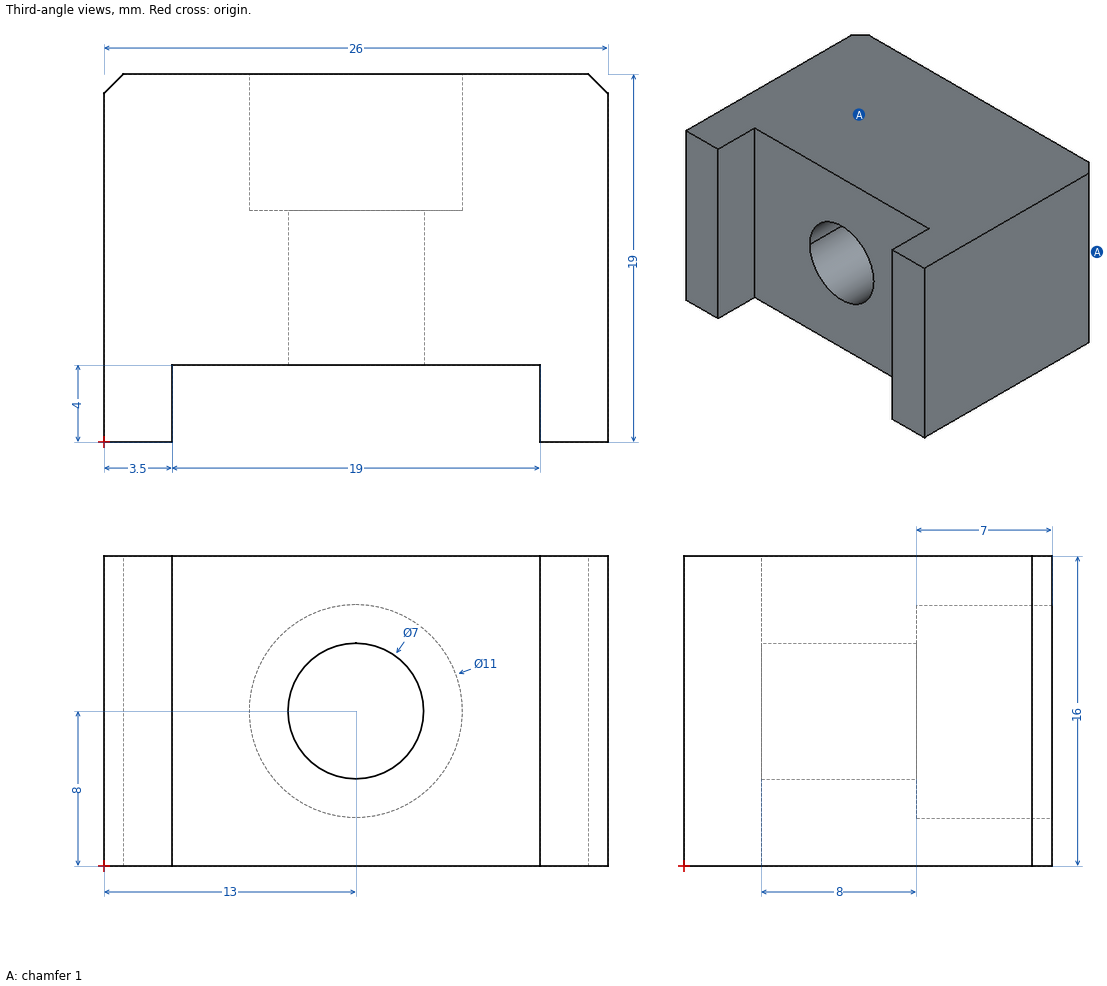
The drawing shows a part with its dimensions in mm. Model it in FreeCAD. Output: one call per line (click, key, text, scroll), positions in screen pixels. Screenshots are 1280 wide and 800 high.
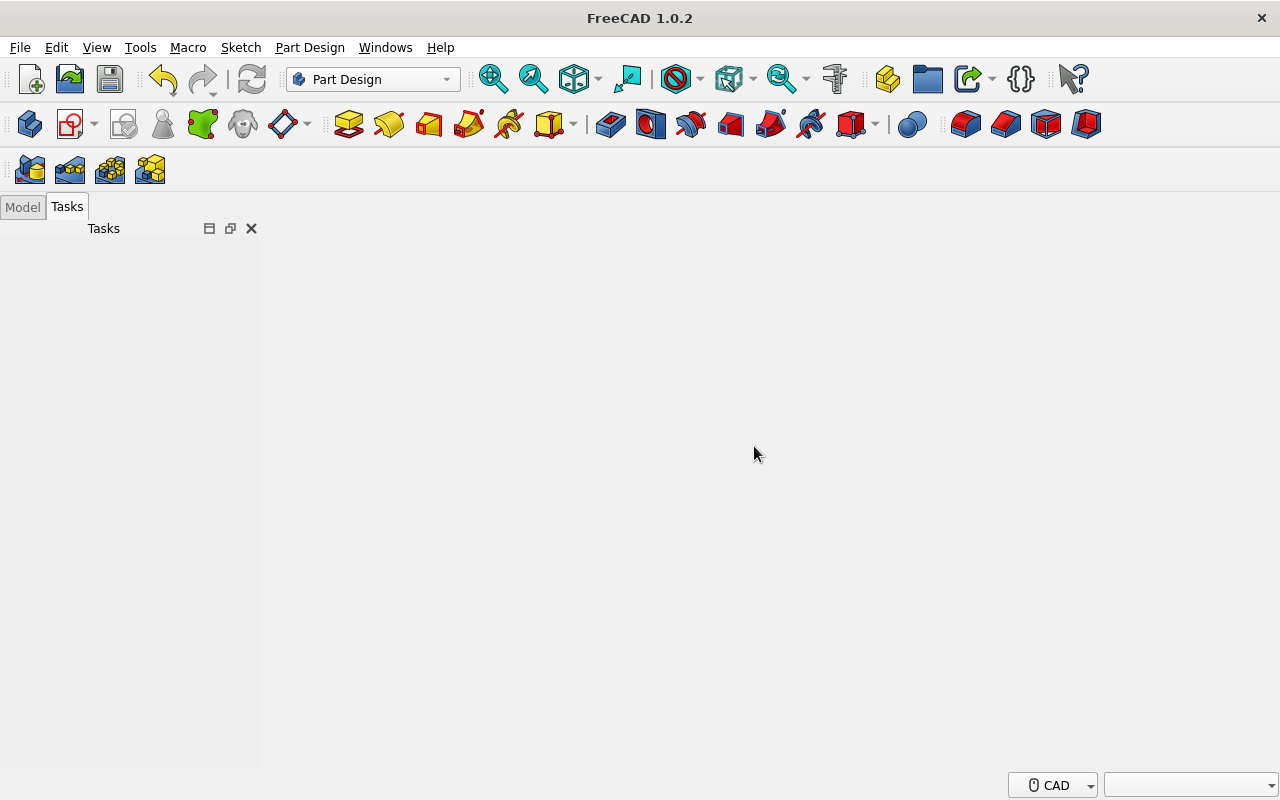
key(ctrl+n)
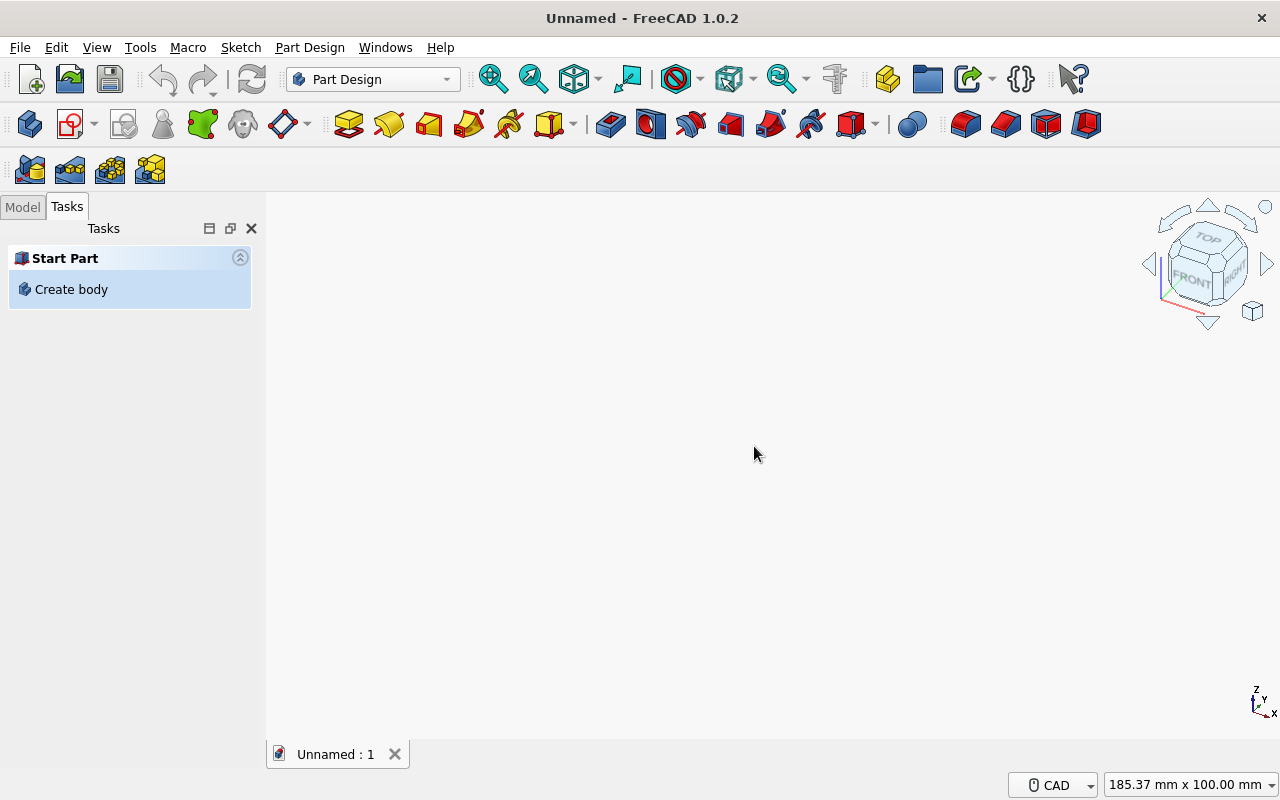
click(70, 124)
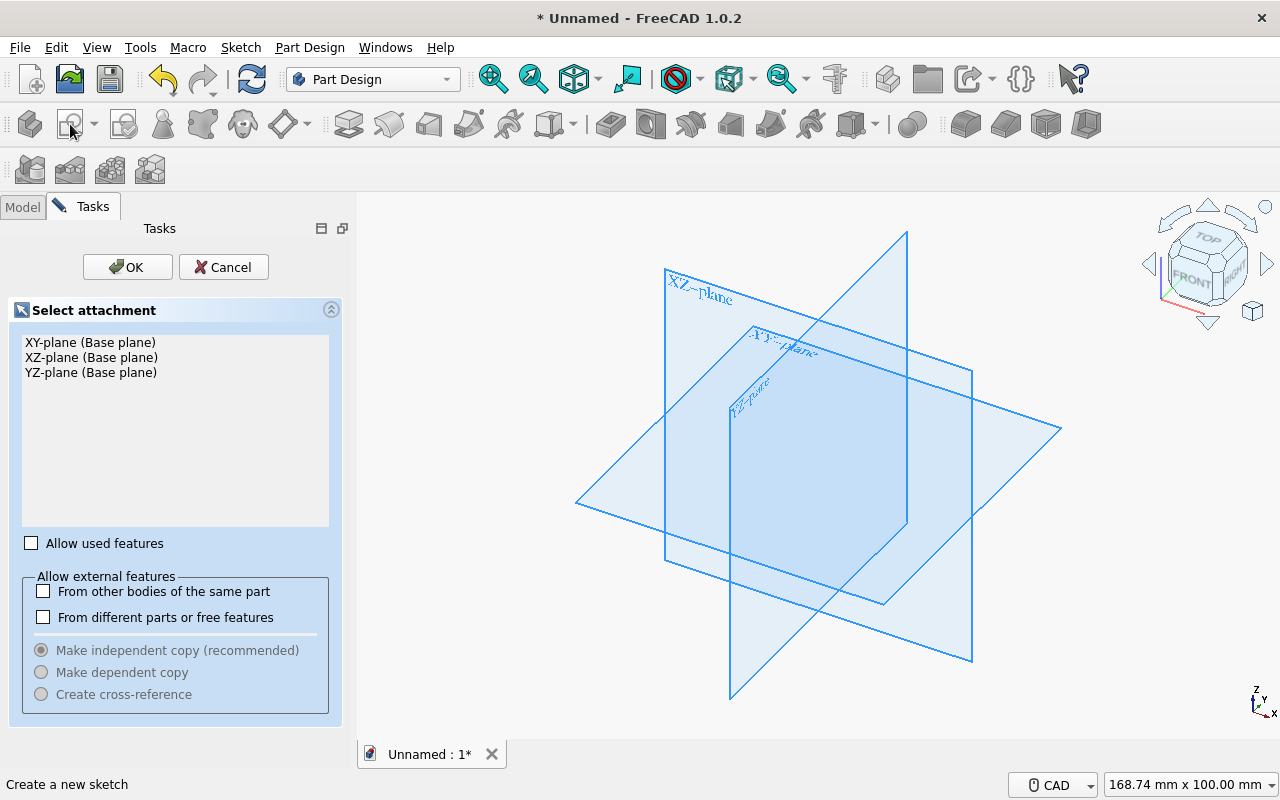
click(82, 342)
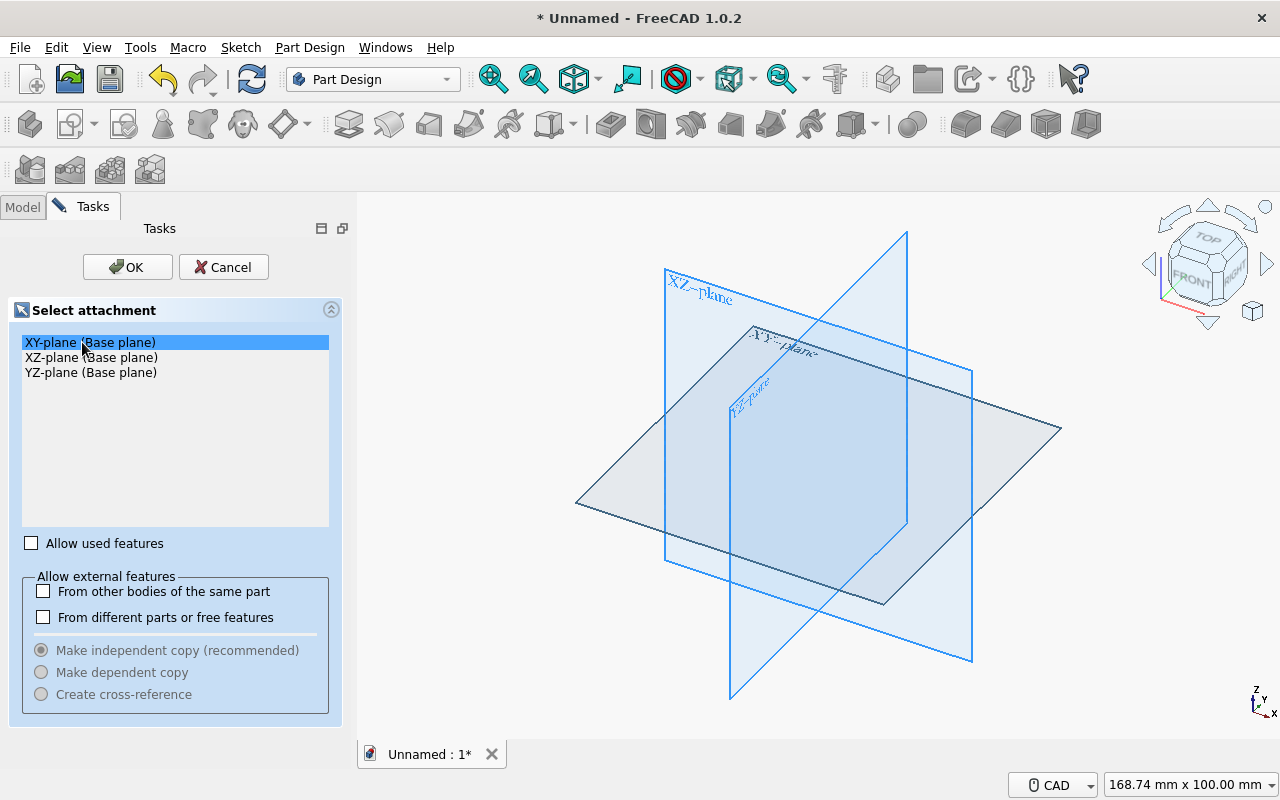
click(128, 267)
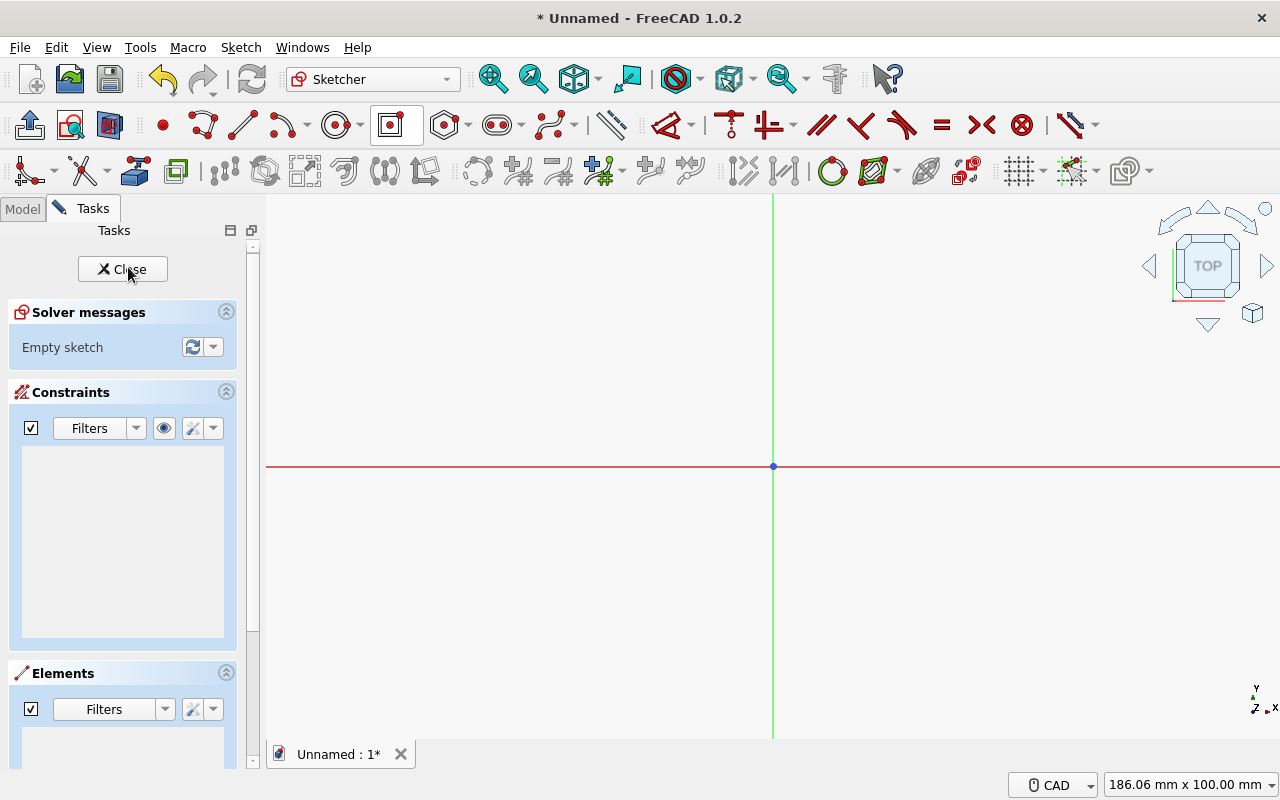
scroll(904, 392, up, 6)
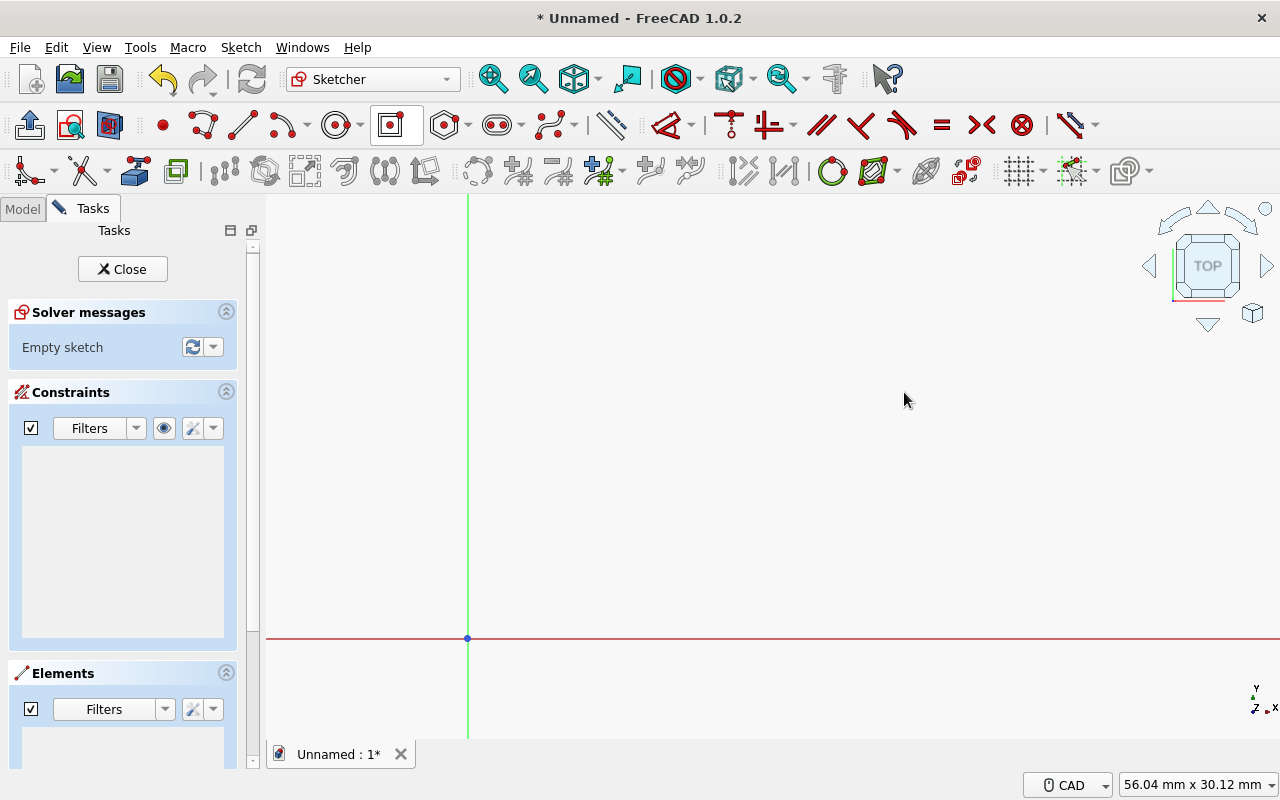
click(204, 126)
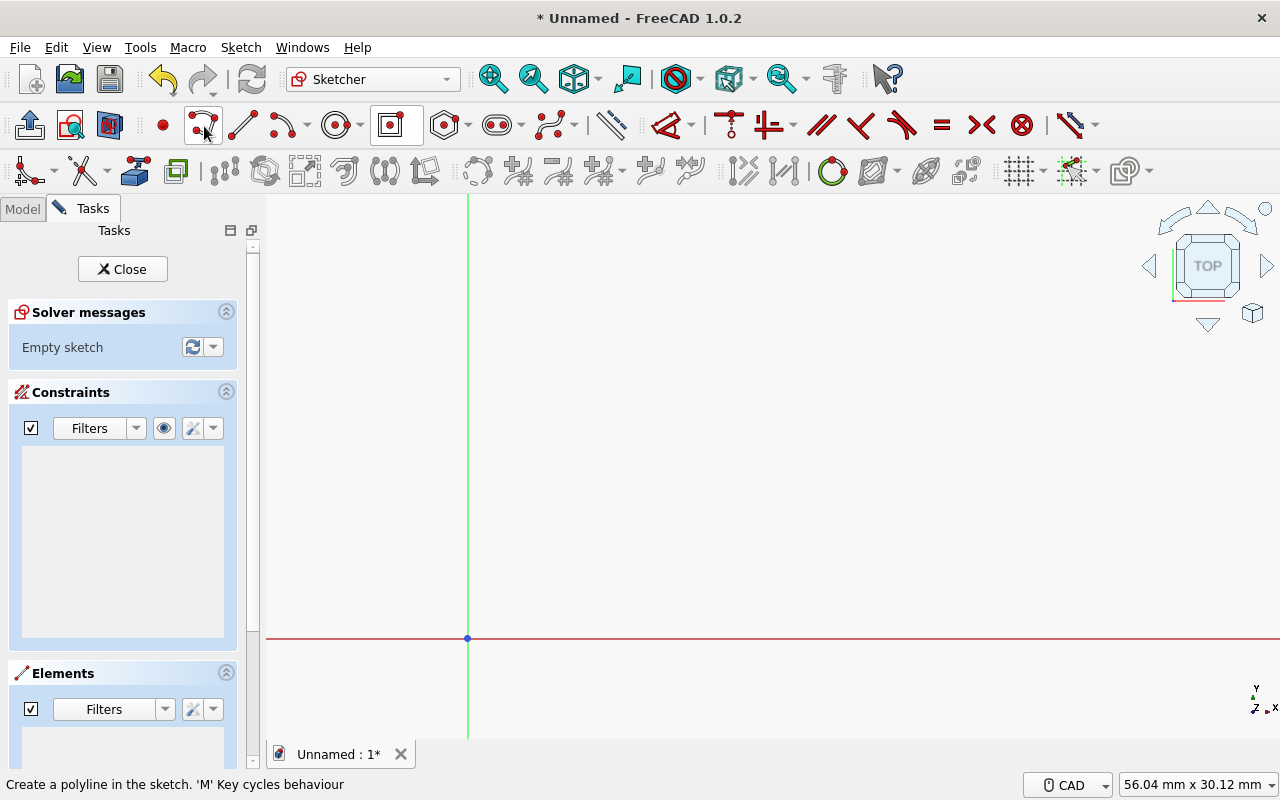
click(468, 639)
click(531, 630)
click(531, 566)
click(875, 566)
click(875, 639)
click(938, 630)
click(938, 295)
click(477, 295)
click(468, 639)
key(Escape)
key(Escape)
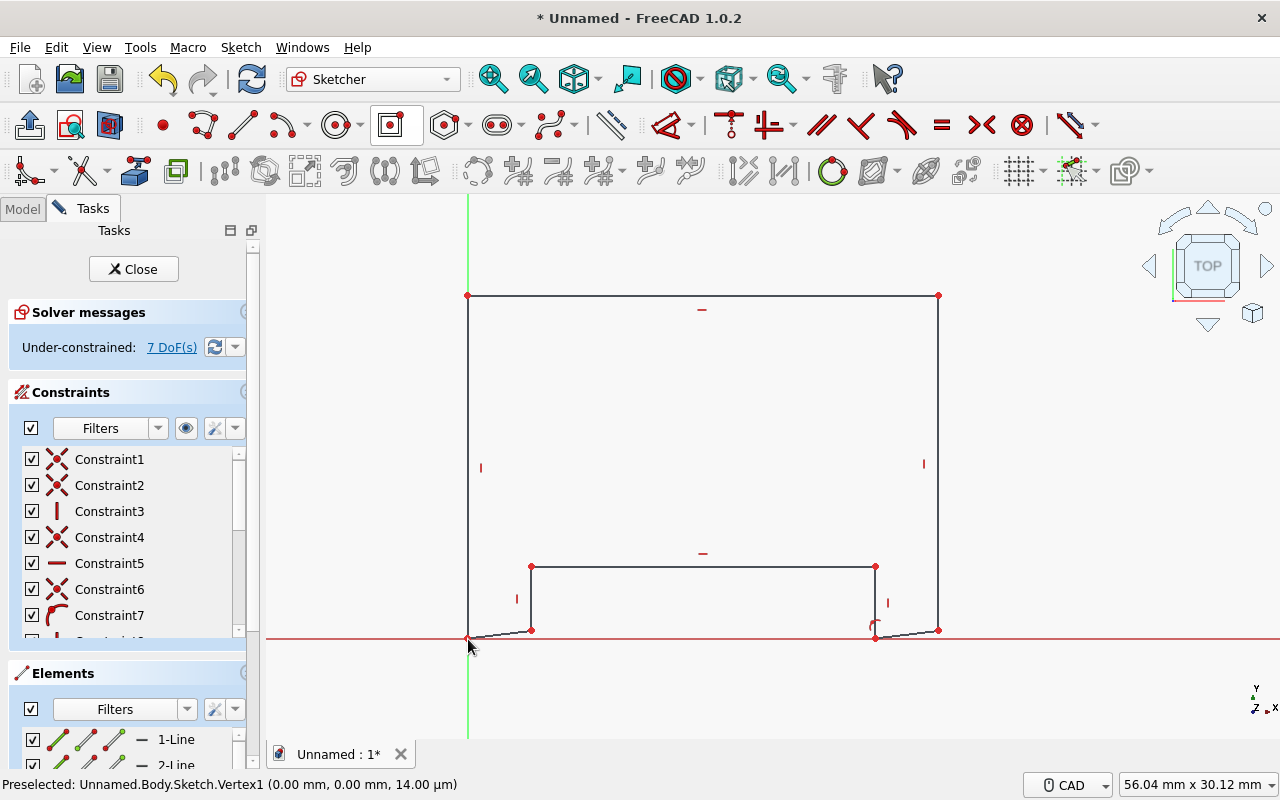
click(487, 636)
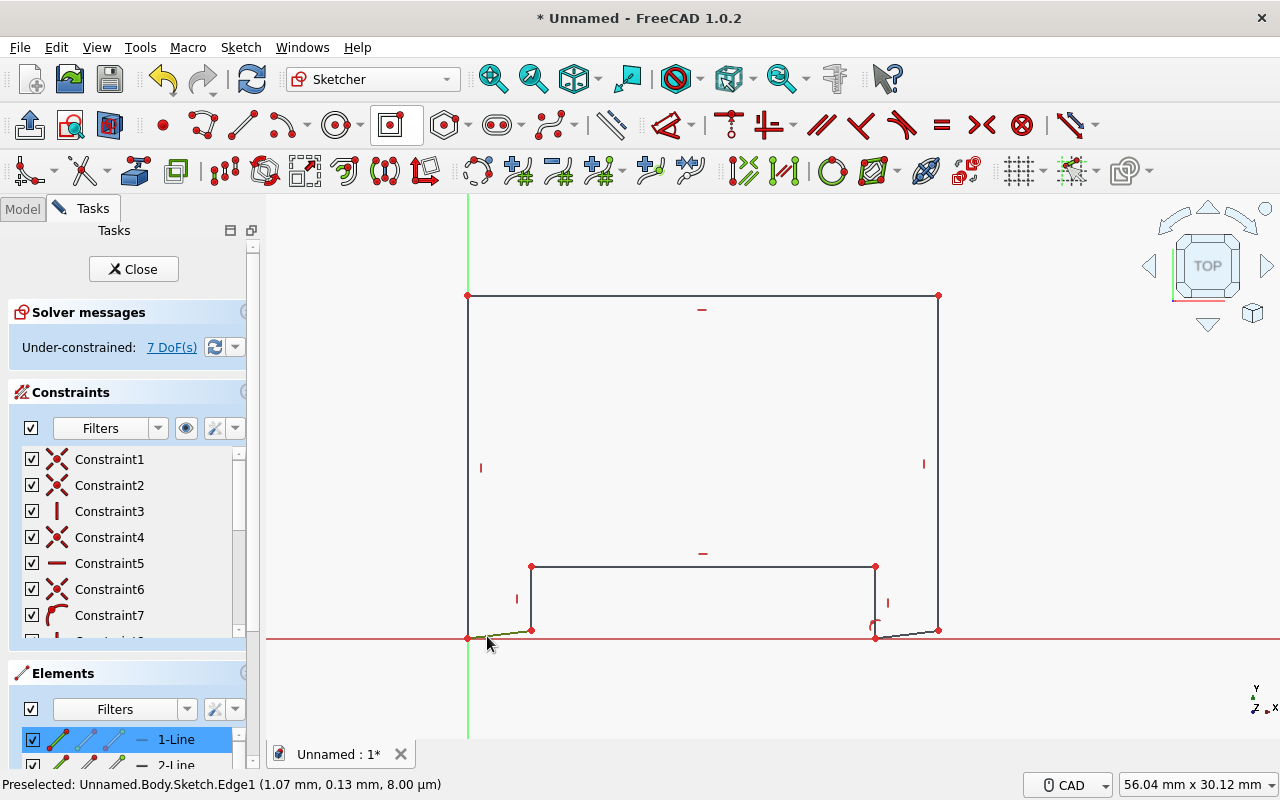
key(h)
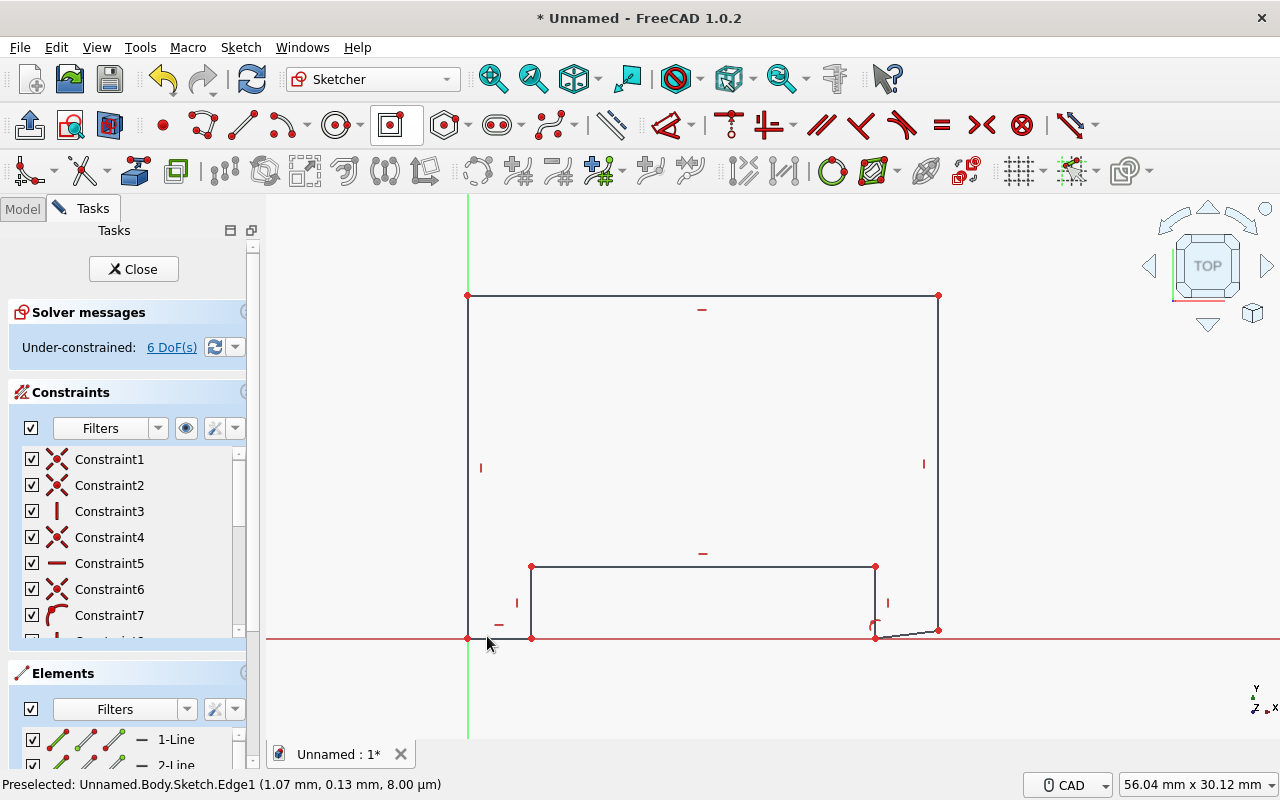
click(894, 636)